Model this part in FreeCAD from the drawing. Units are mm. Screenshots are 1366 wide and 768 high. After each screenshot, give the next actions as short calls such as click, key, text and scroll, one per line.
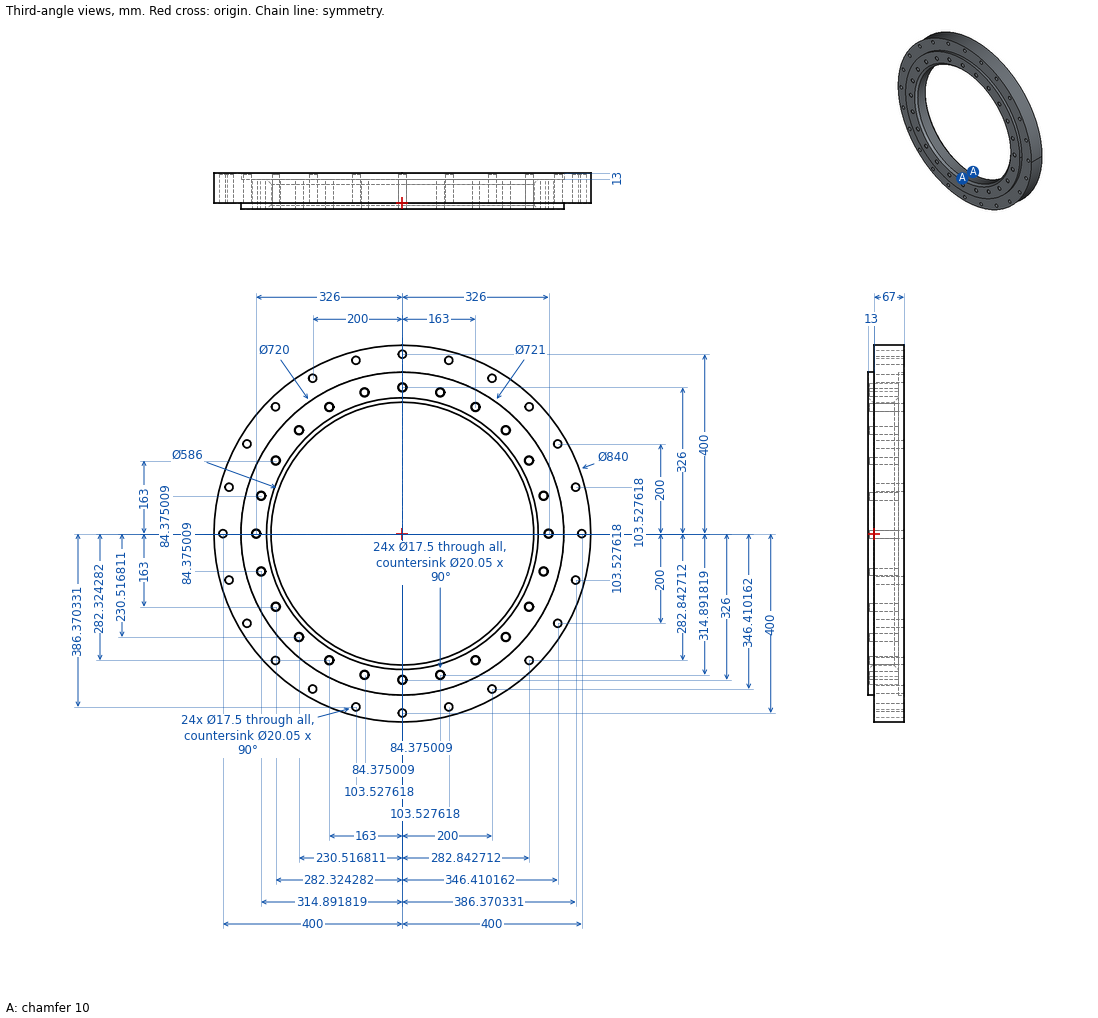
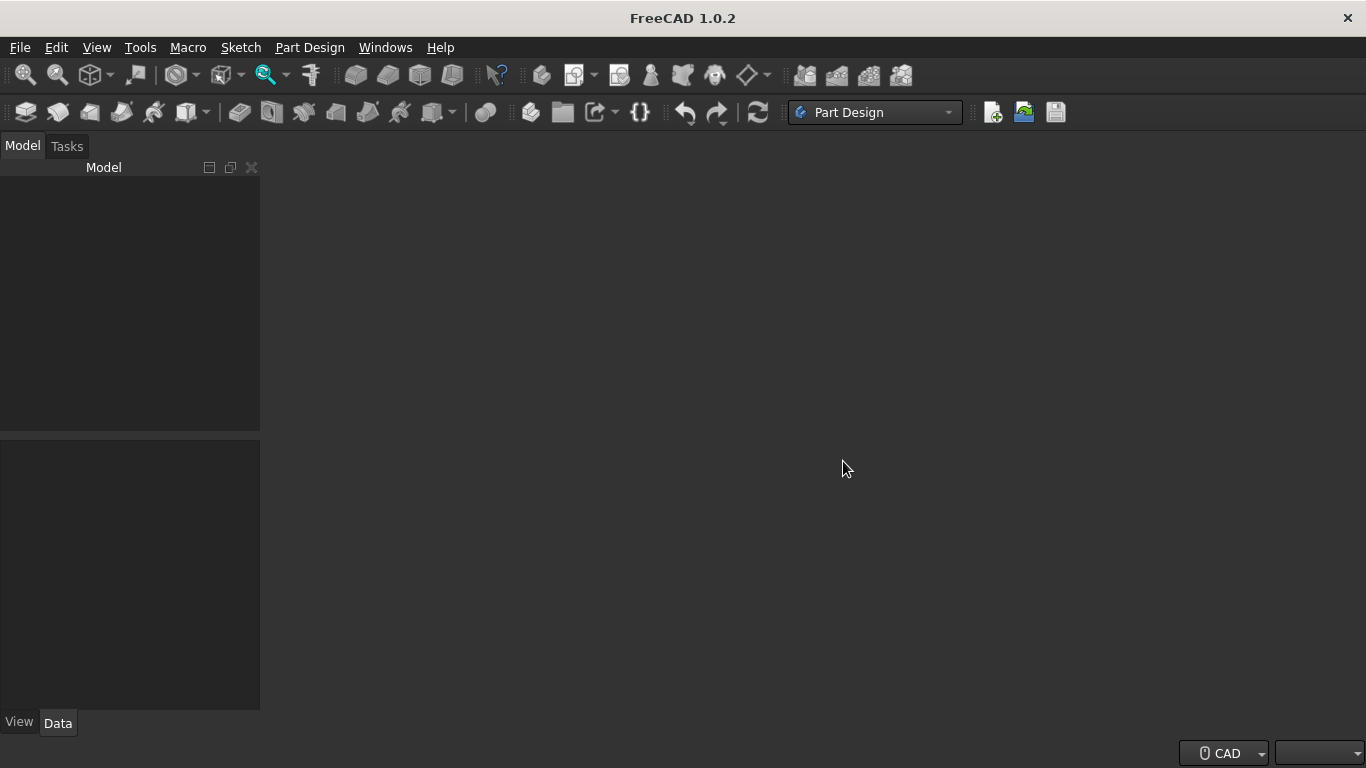
click(992, 112)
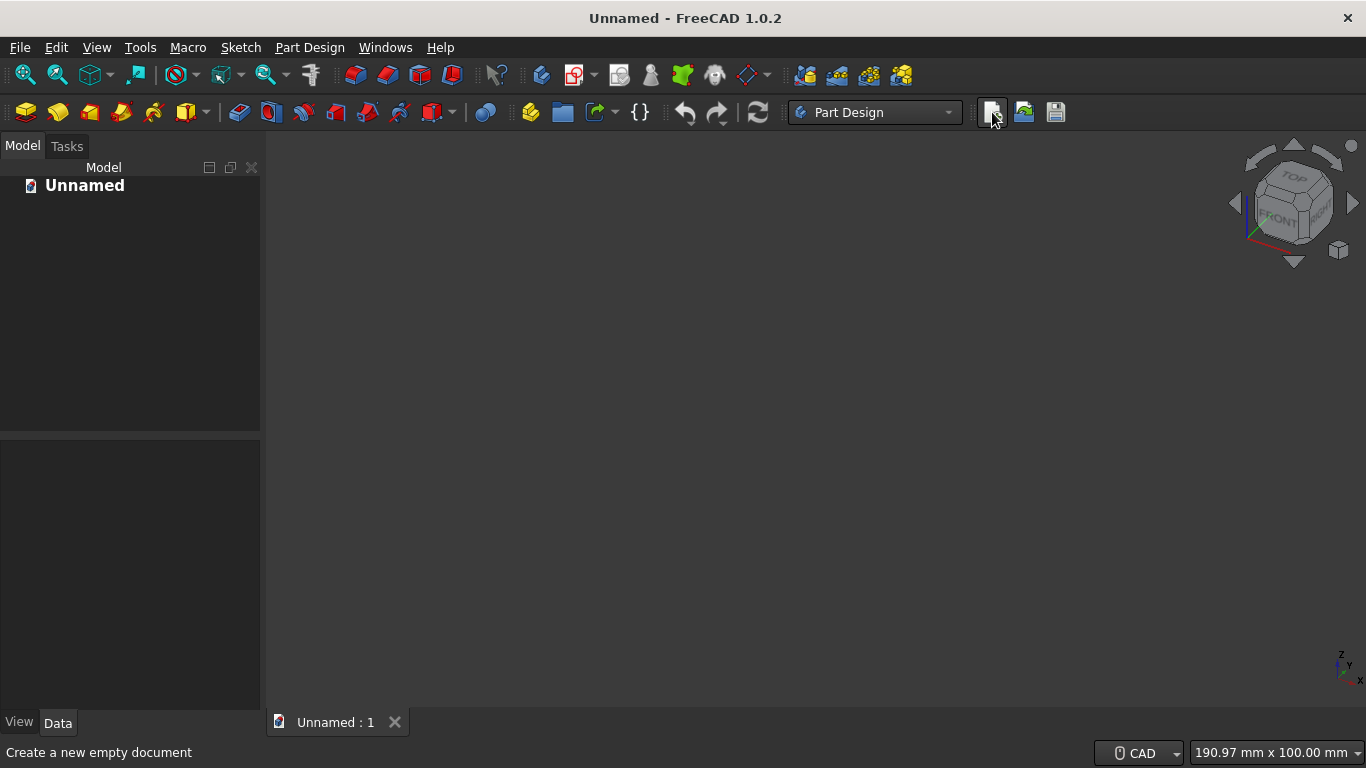
click(574, 76)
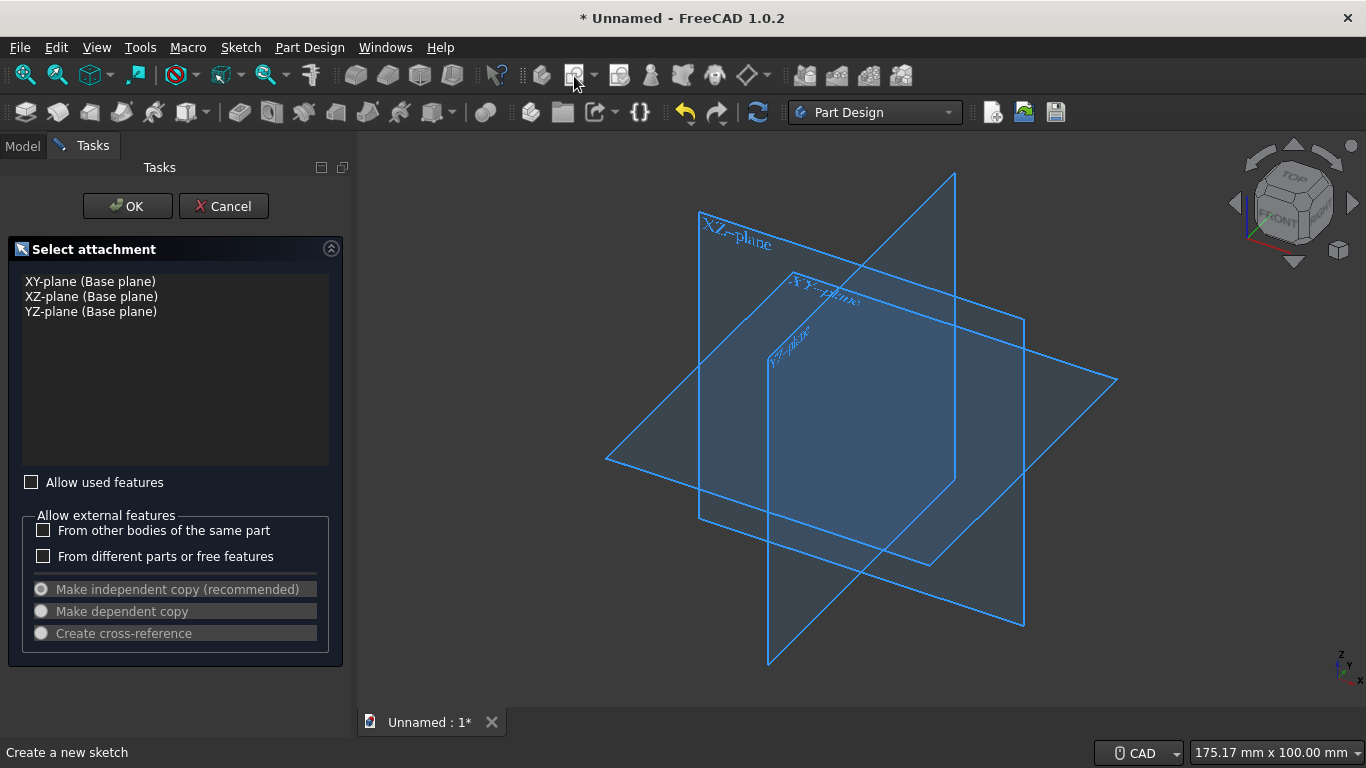
click(82, 296)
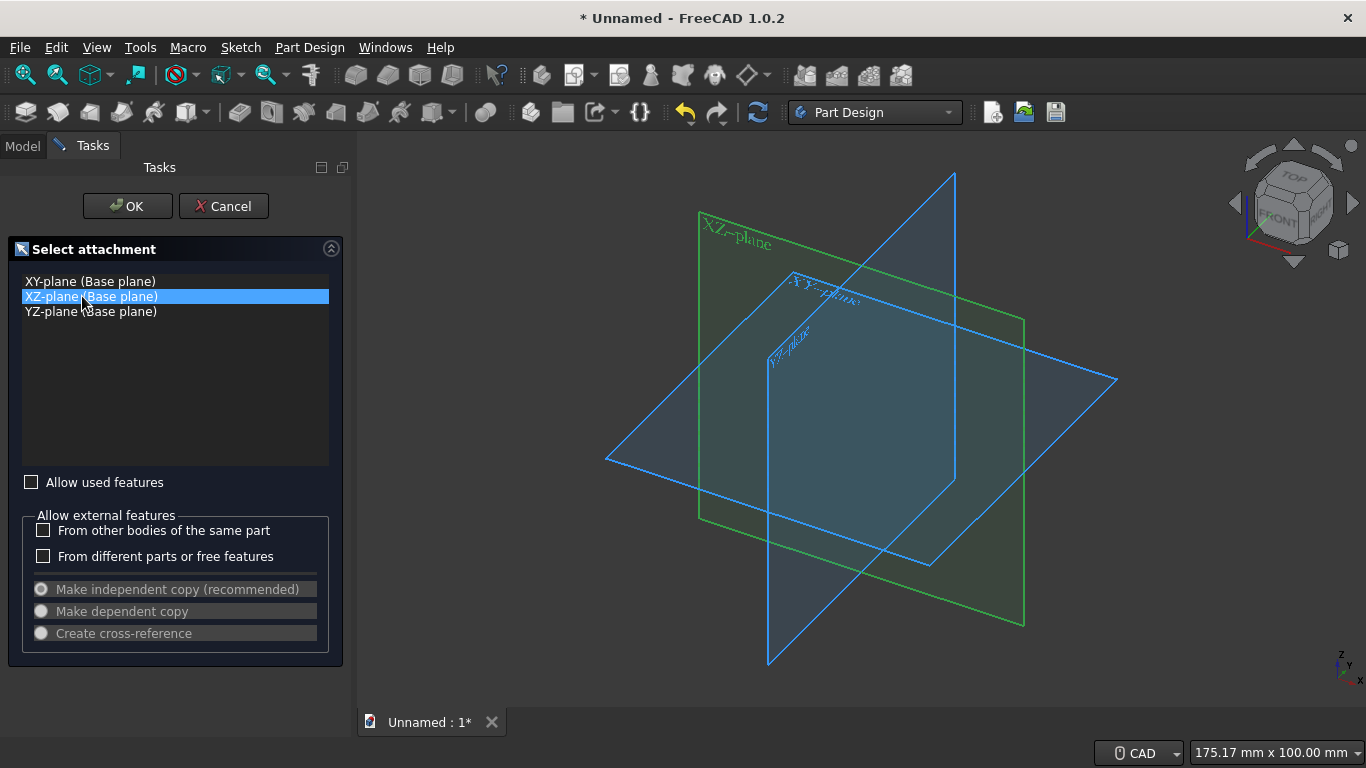
click(128, 206)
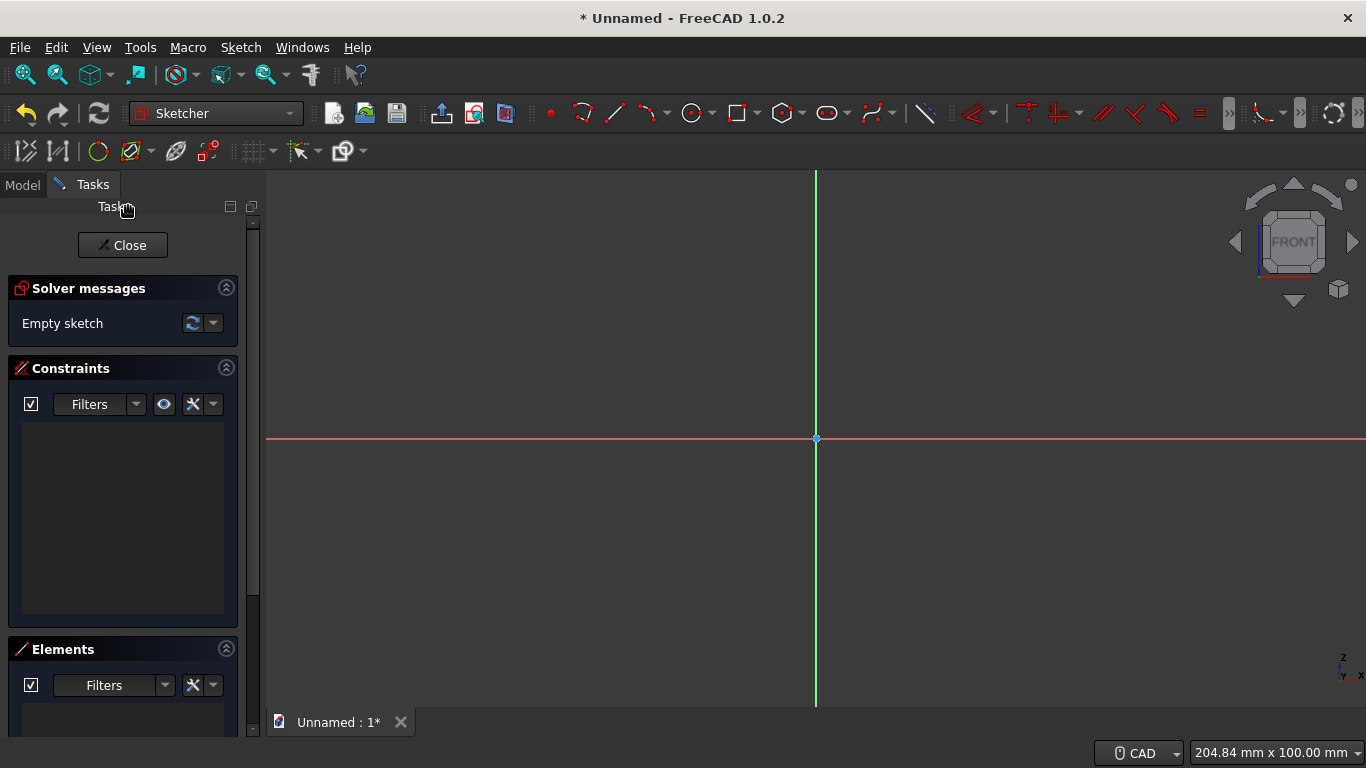
scroll(742, 438, down, 13)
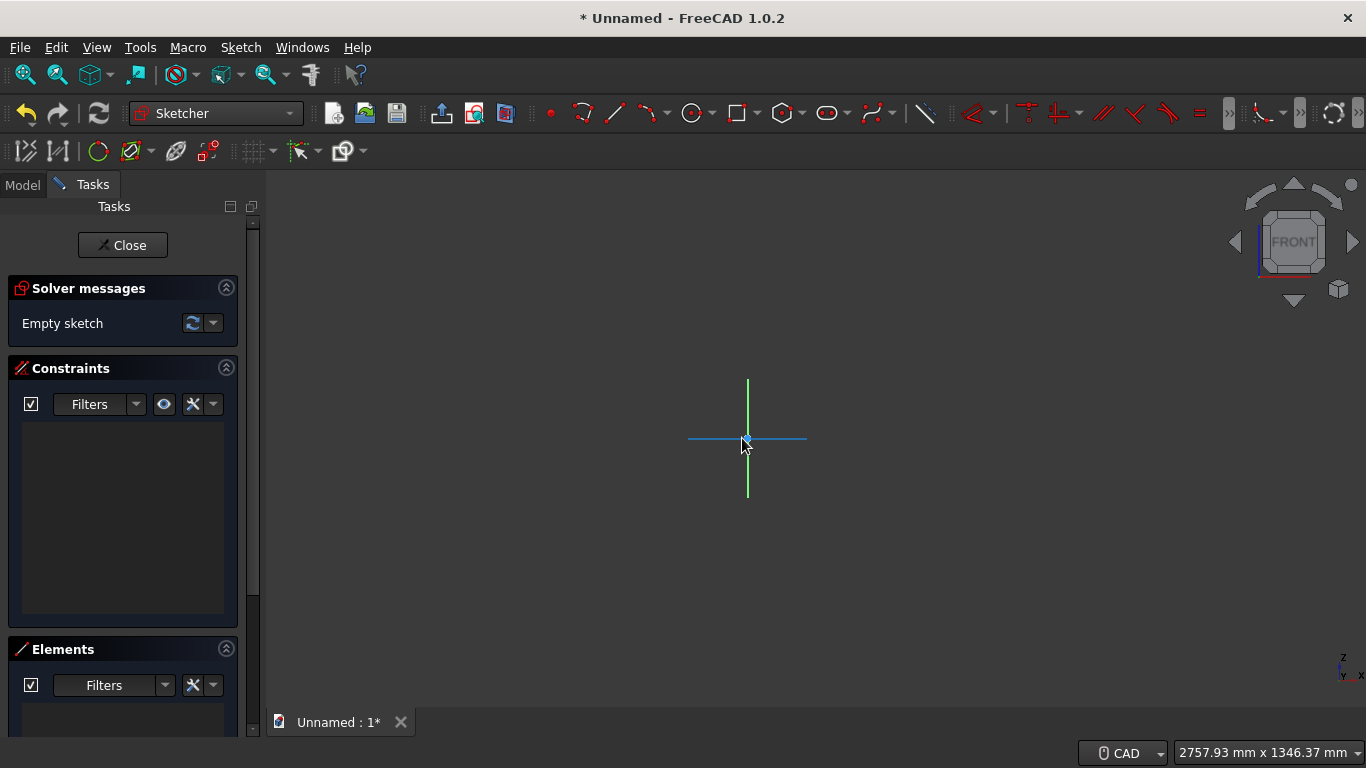
key(g)
key(c)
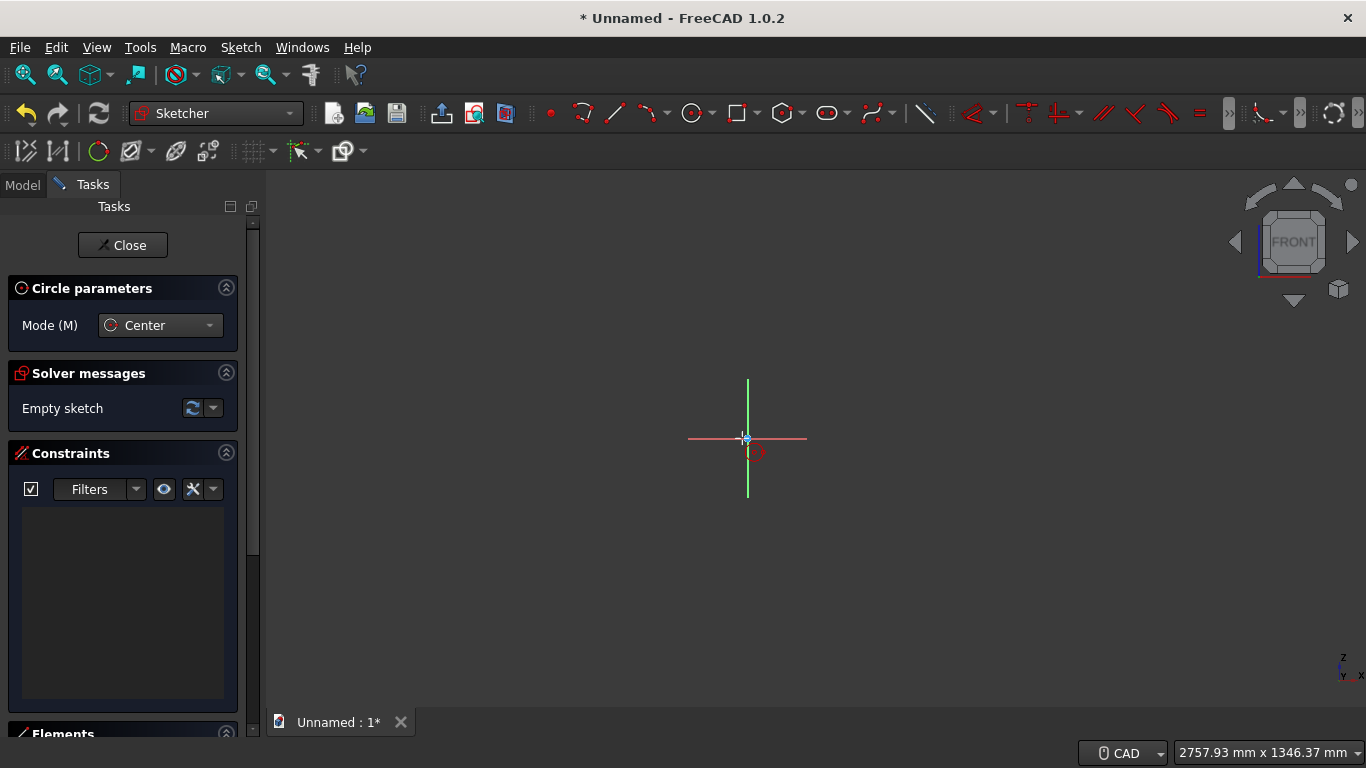
click(748, 438)
click(866, 320)
key(Escape)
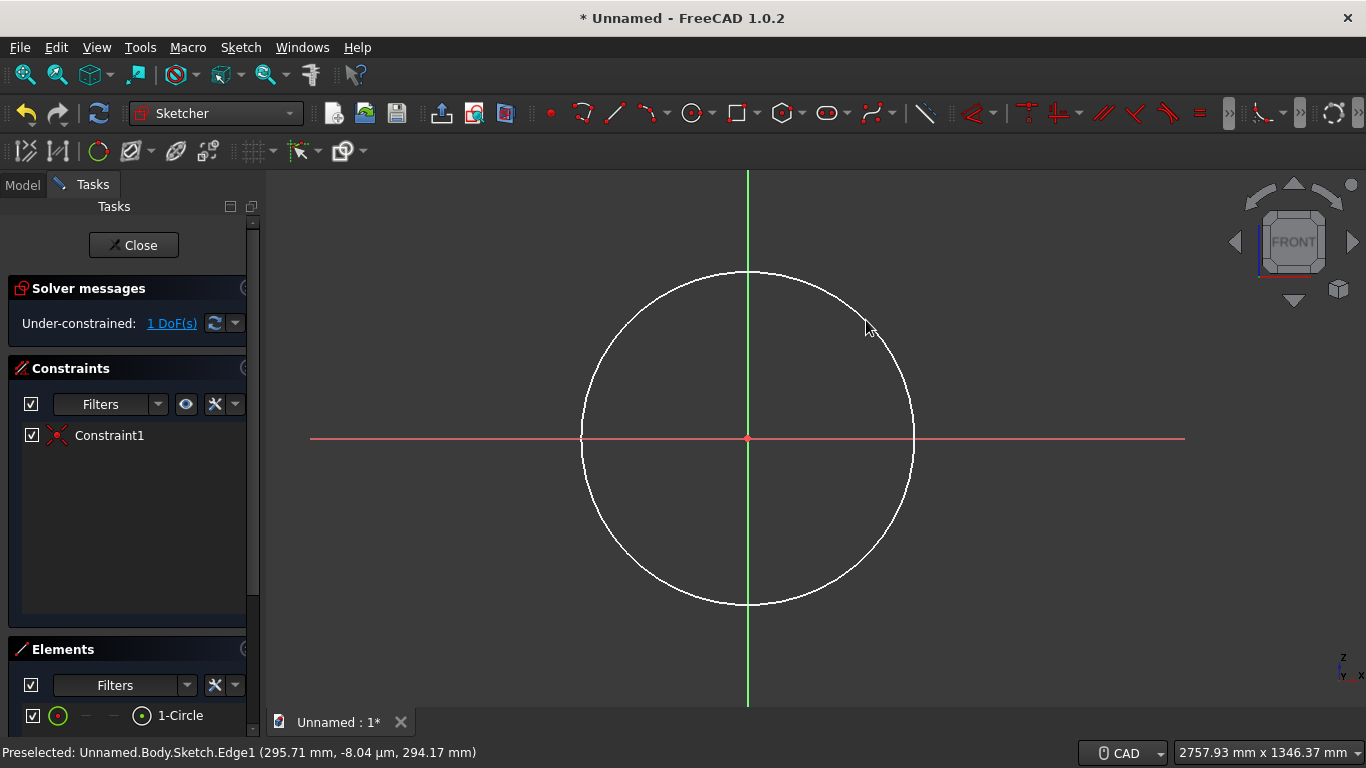
click(865, 320)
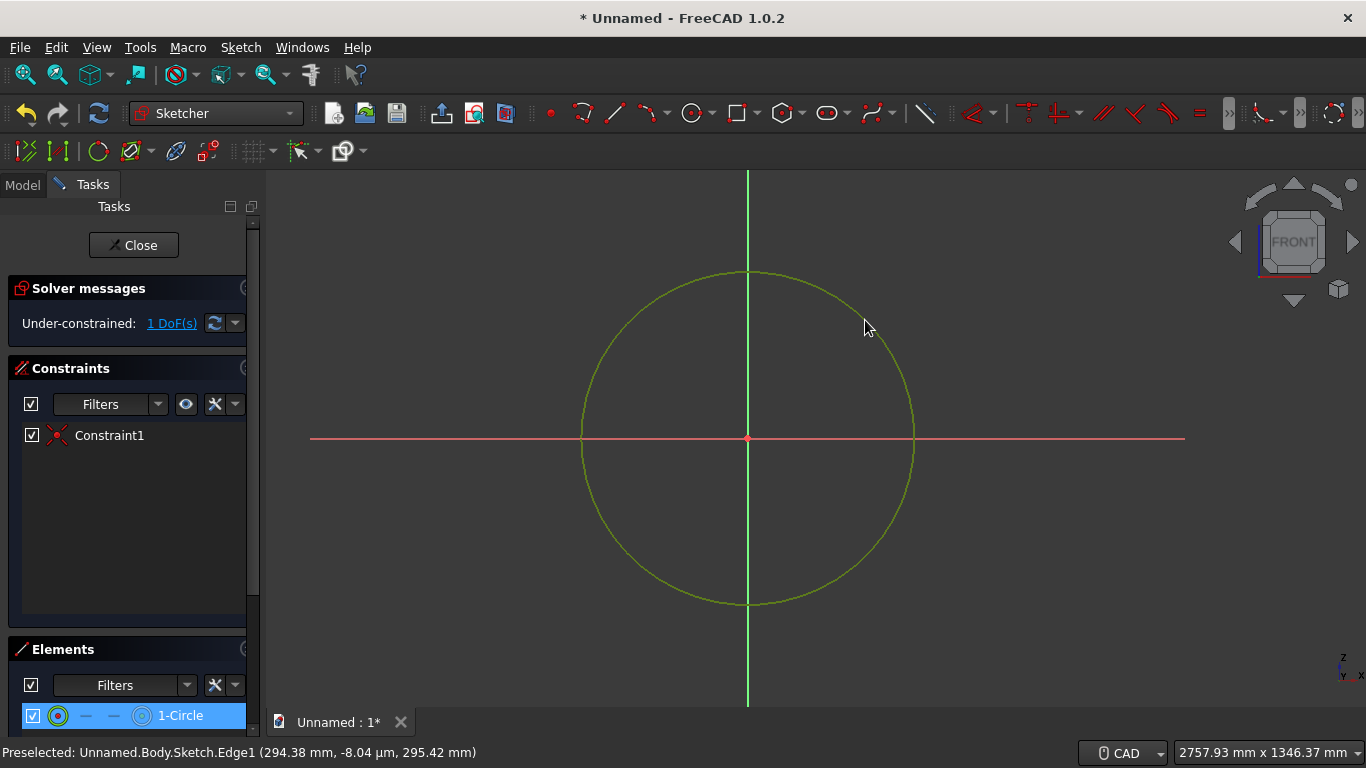
key(k)
key(o)